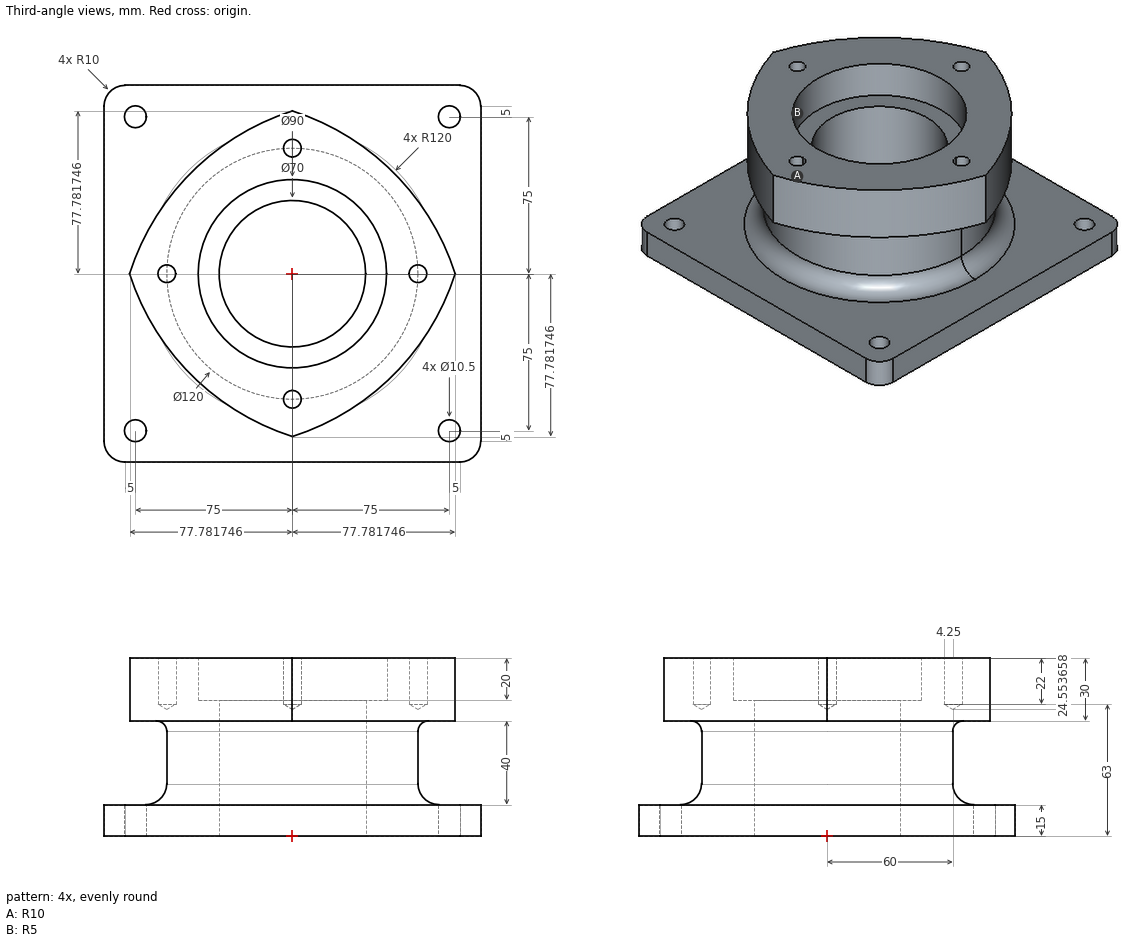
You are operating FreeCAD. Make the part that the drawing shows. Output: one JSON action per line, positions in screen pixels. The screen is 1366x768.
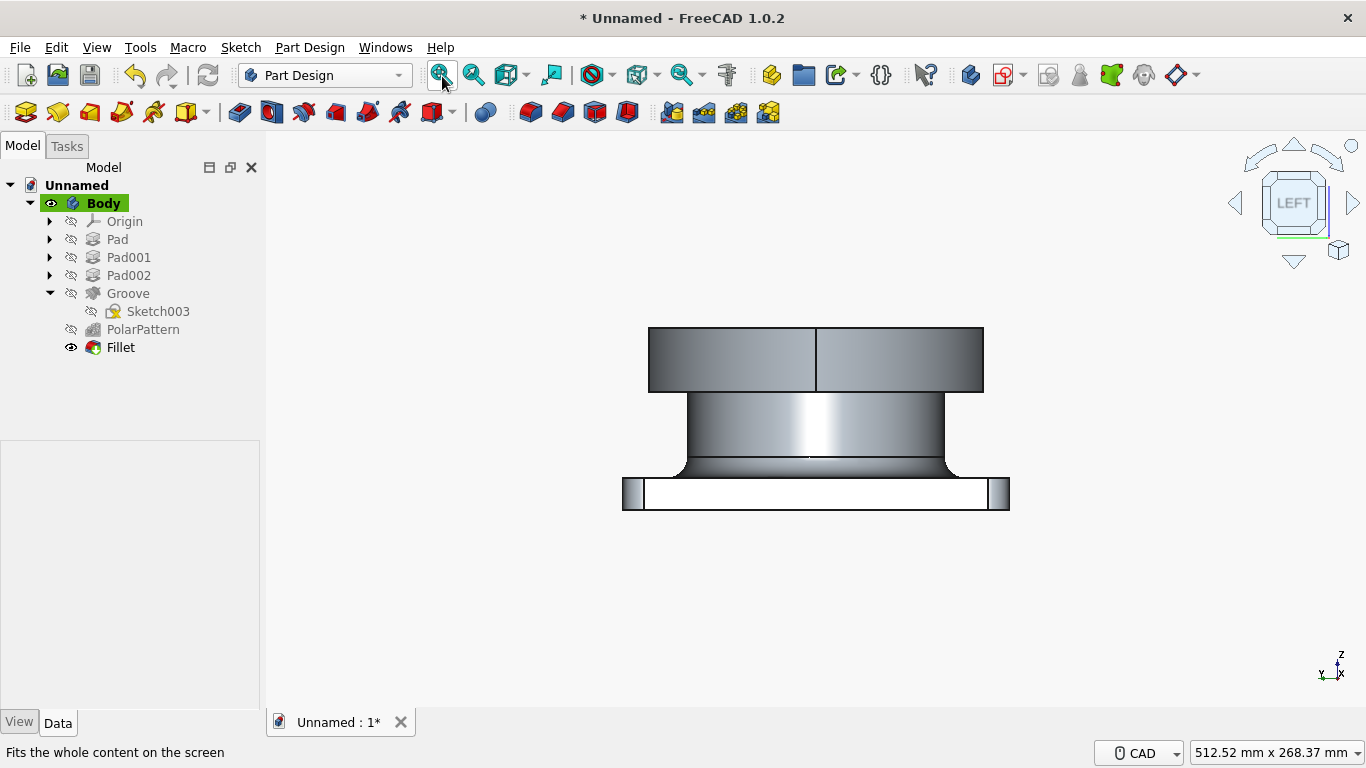
{"action": "left_click", "coordinate": [442, 76]}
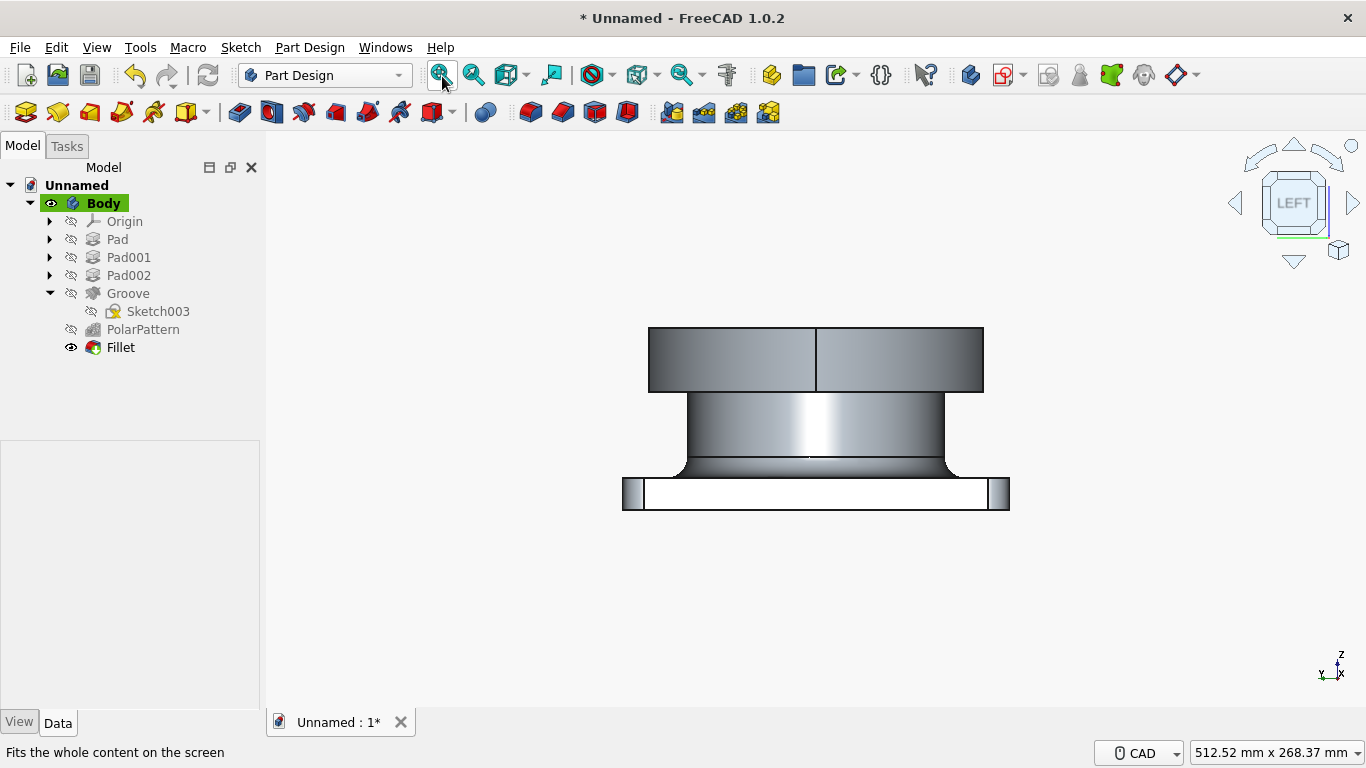
{"action": "key", "text": "v 3"}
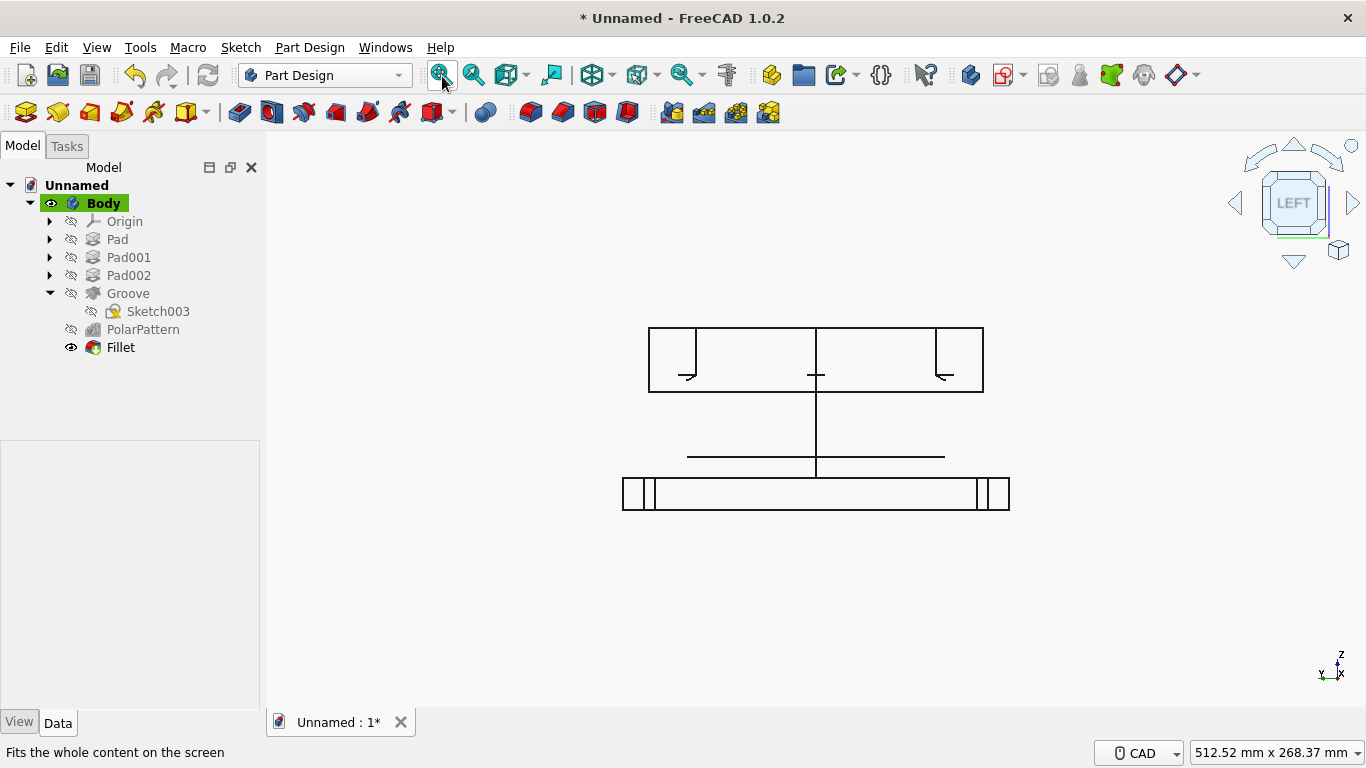
{"action": "key", "text": "0"}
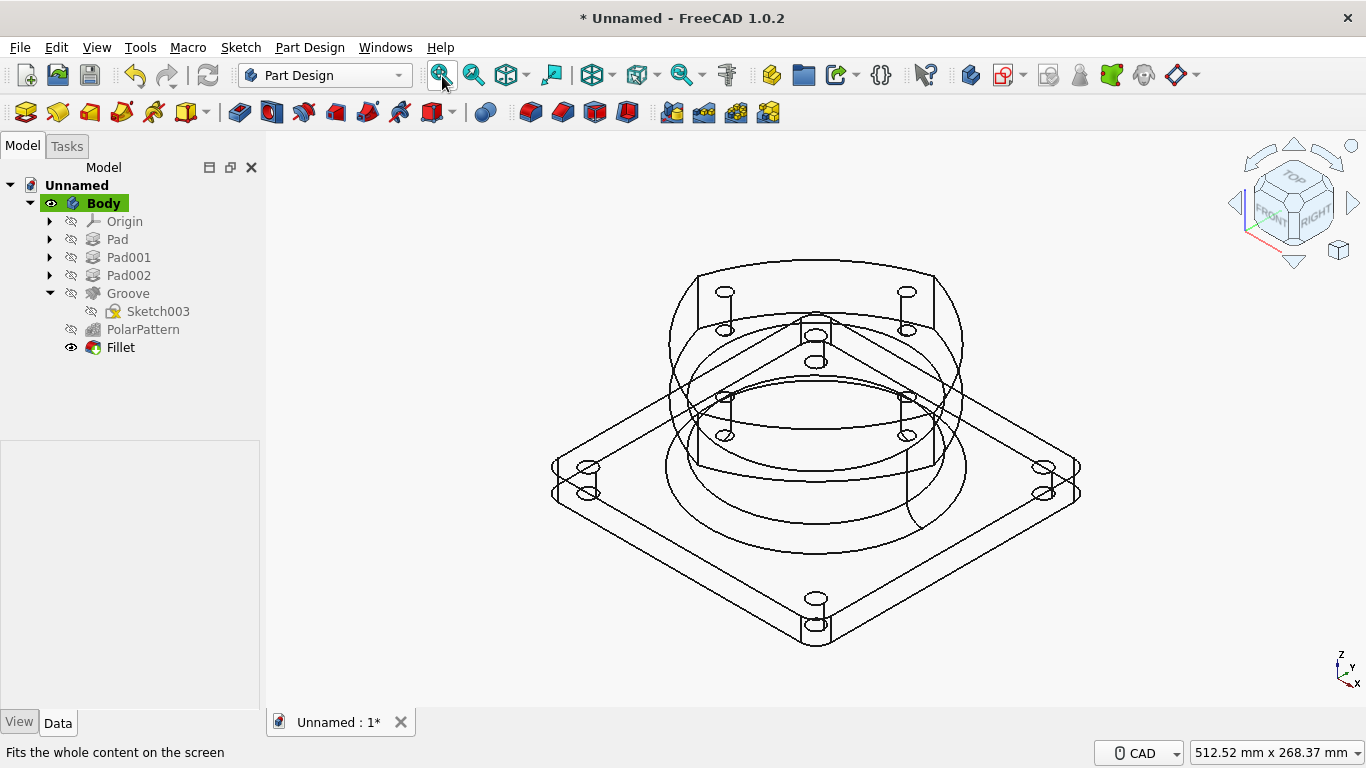
{"action": "left_click", "coordinate": [725, 344]}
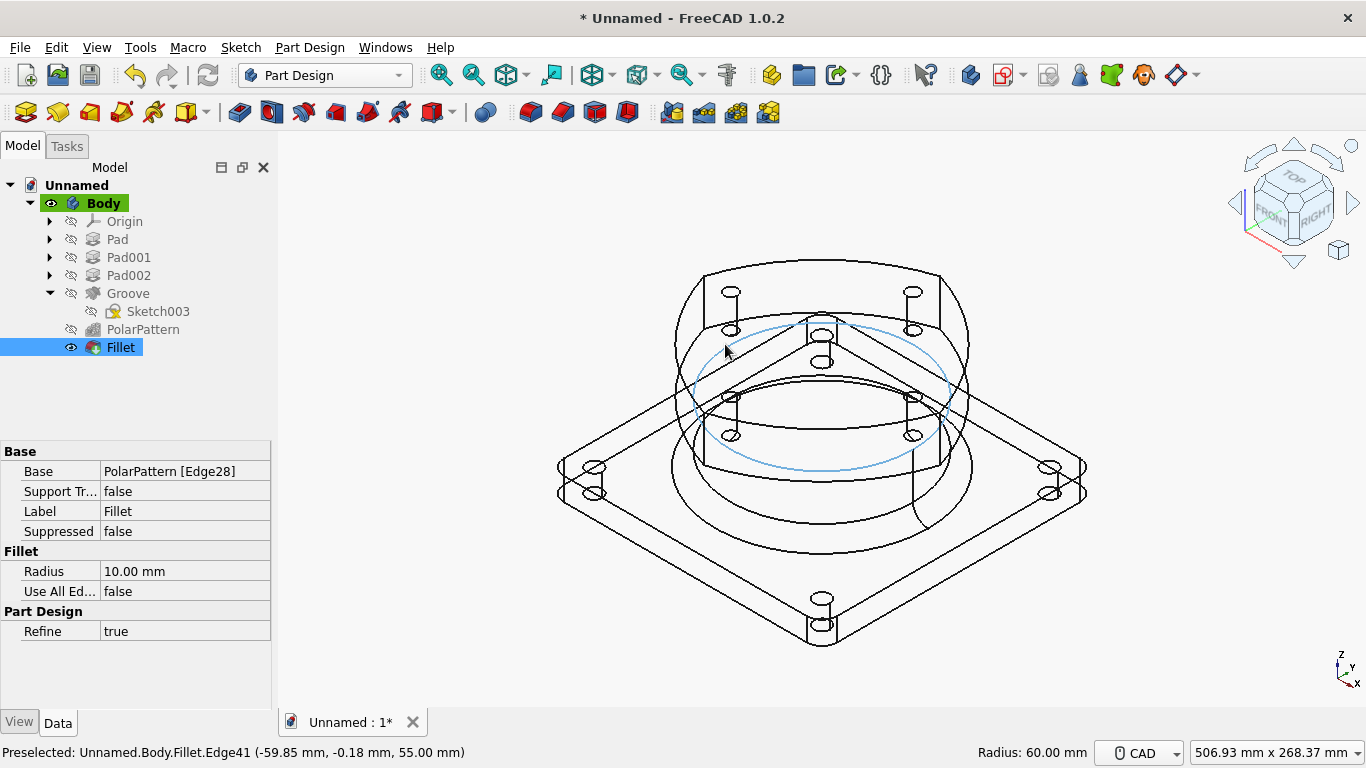
{"action": "key", "text": "v 1"}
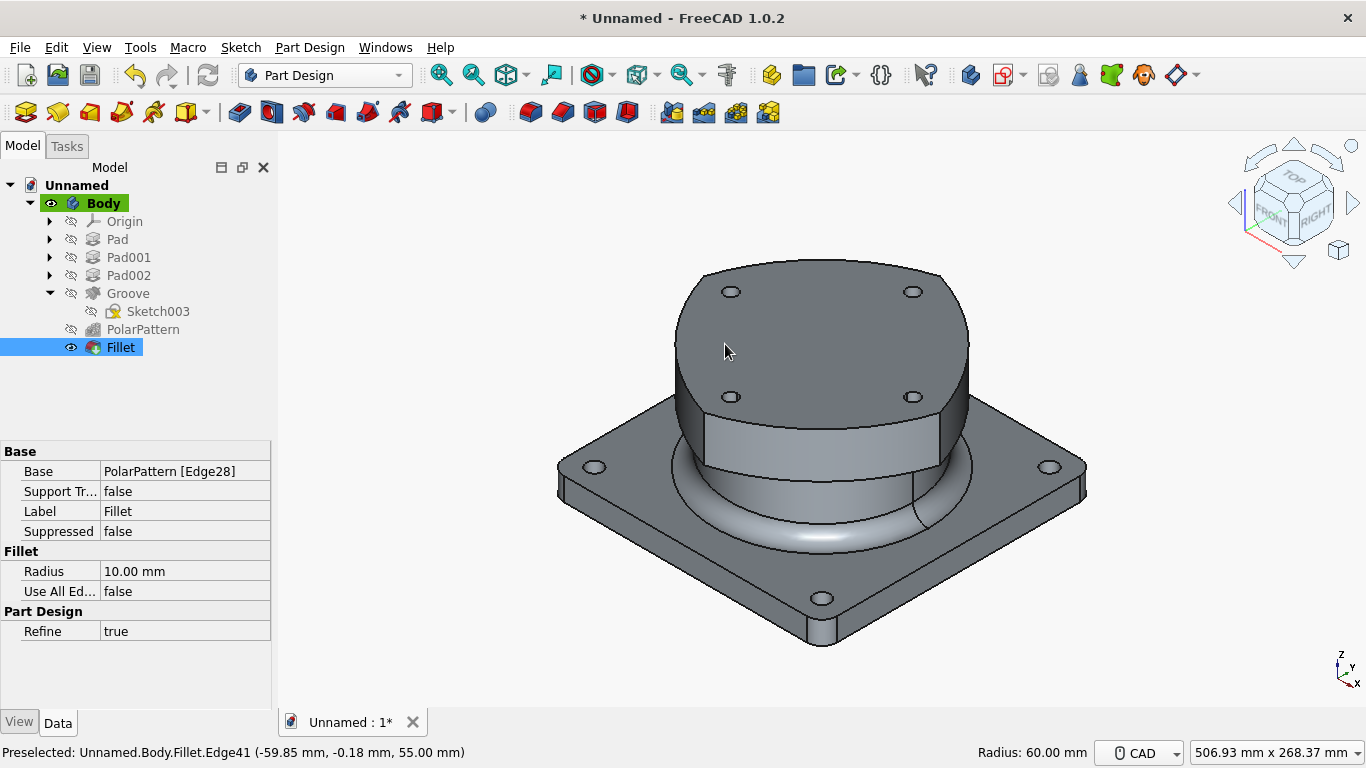
{"action": "left_click", "coordinate": [532, 112]}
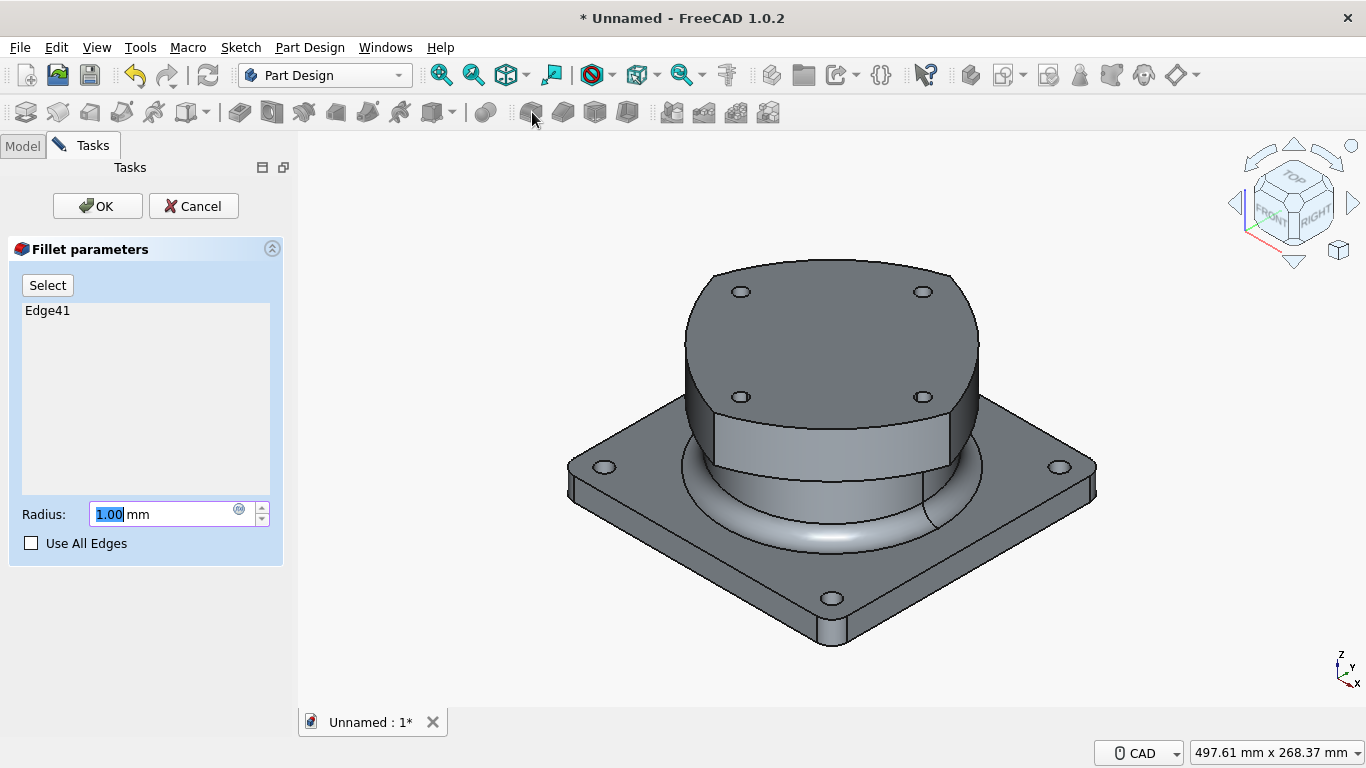
{"action": "type", "text": "5"}
{"action": "key", "text": "Tab"}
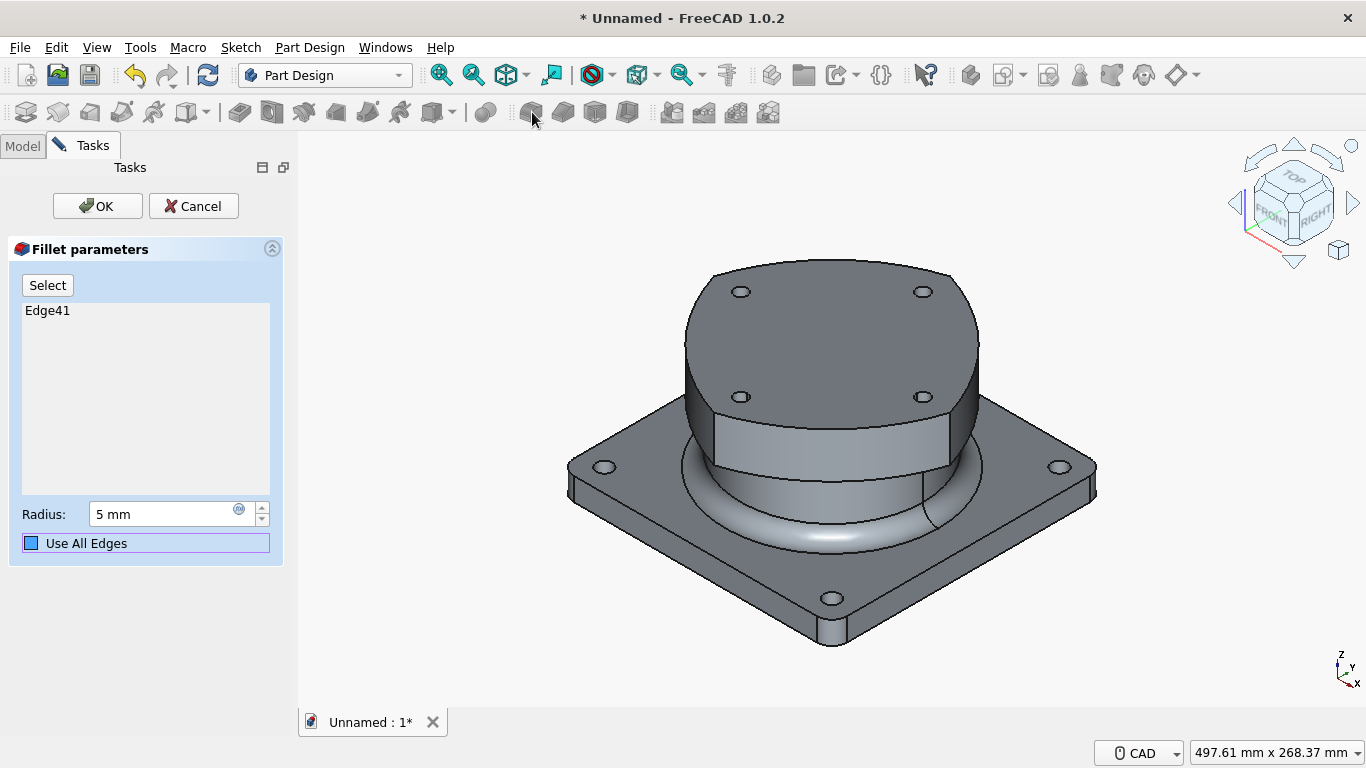
{"action": "left_click", "coordinate": [98, 206]}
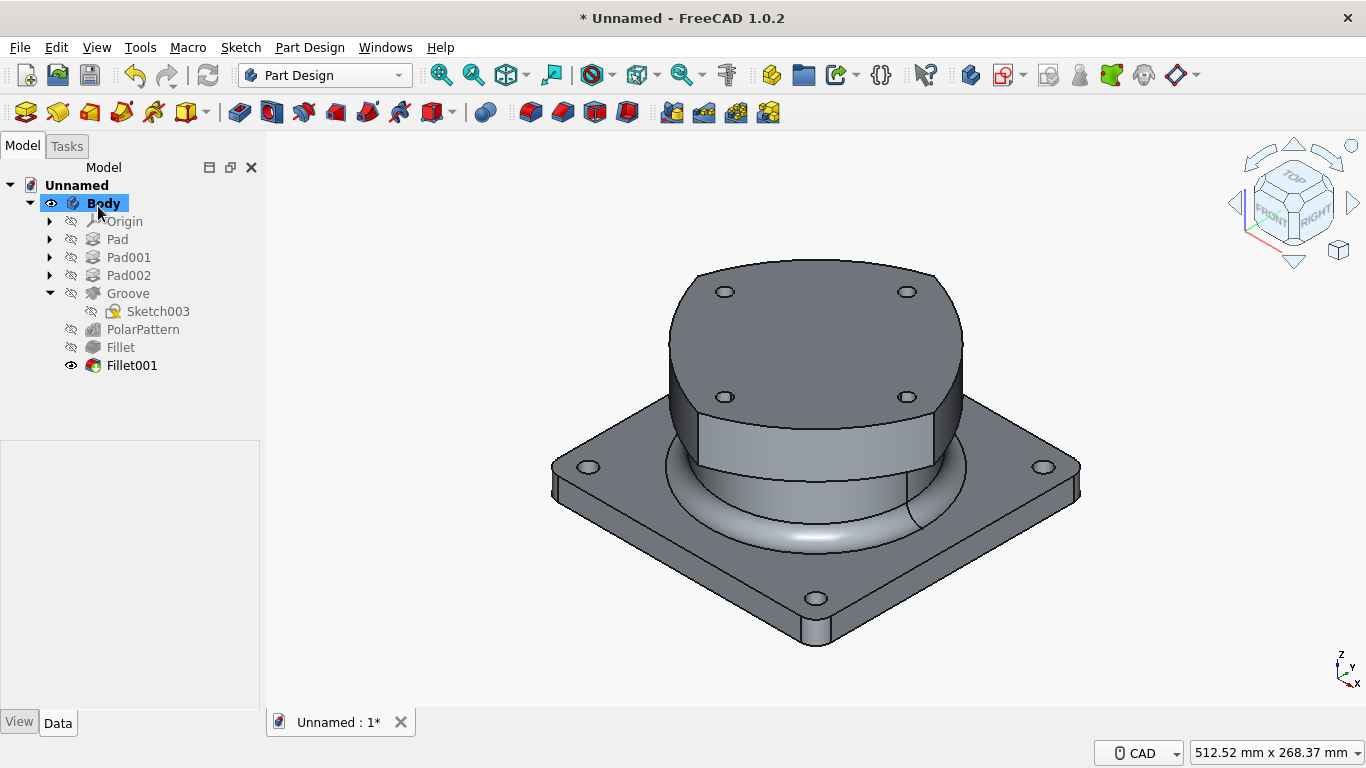
{"action": "left_click", "coordinate": [816, 344]}